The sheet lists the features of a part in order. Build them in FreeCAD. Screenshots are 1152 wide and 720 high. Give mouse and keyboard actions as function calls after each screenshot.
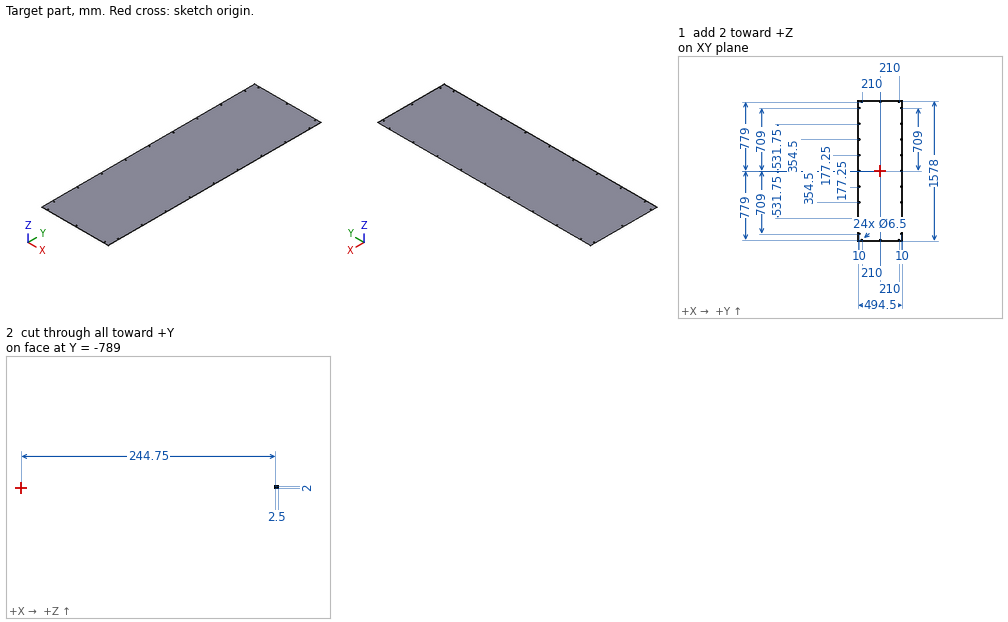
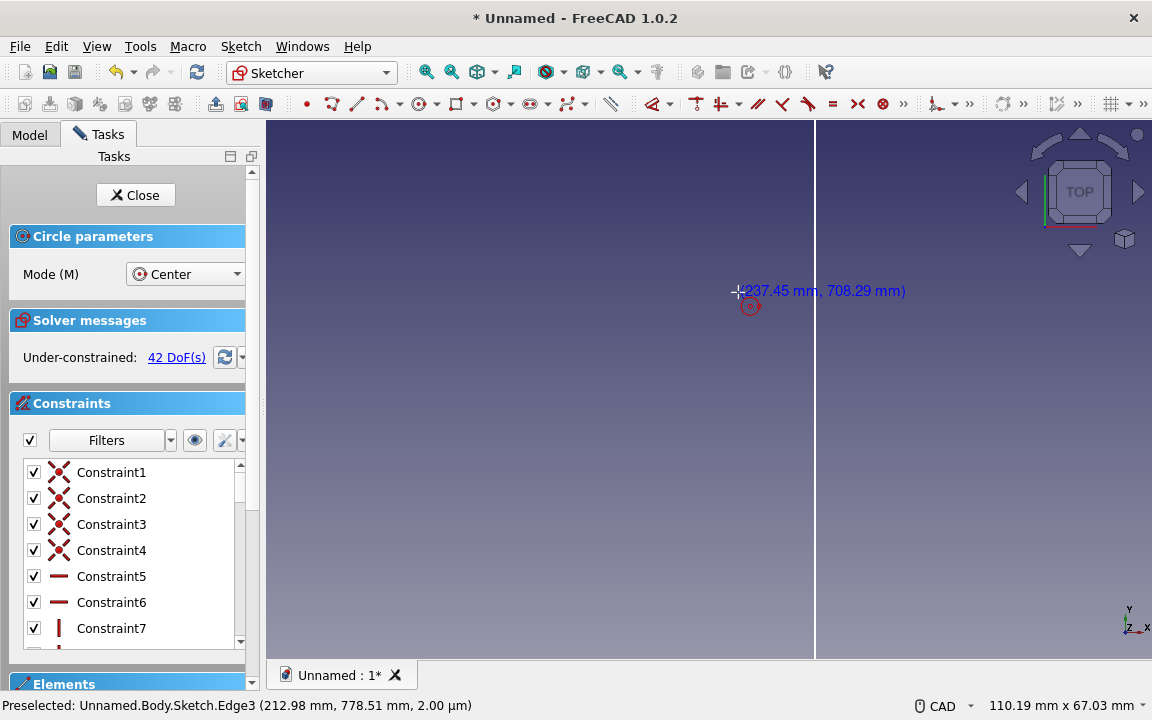
scroll(703, 196, down, 17)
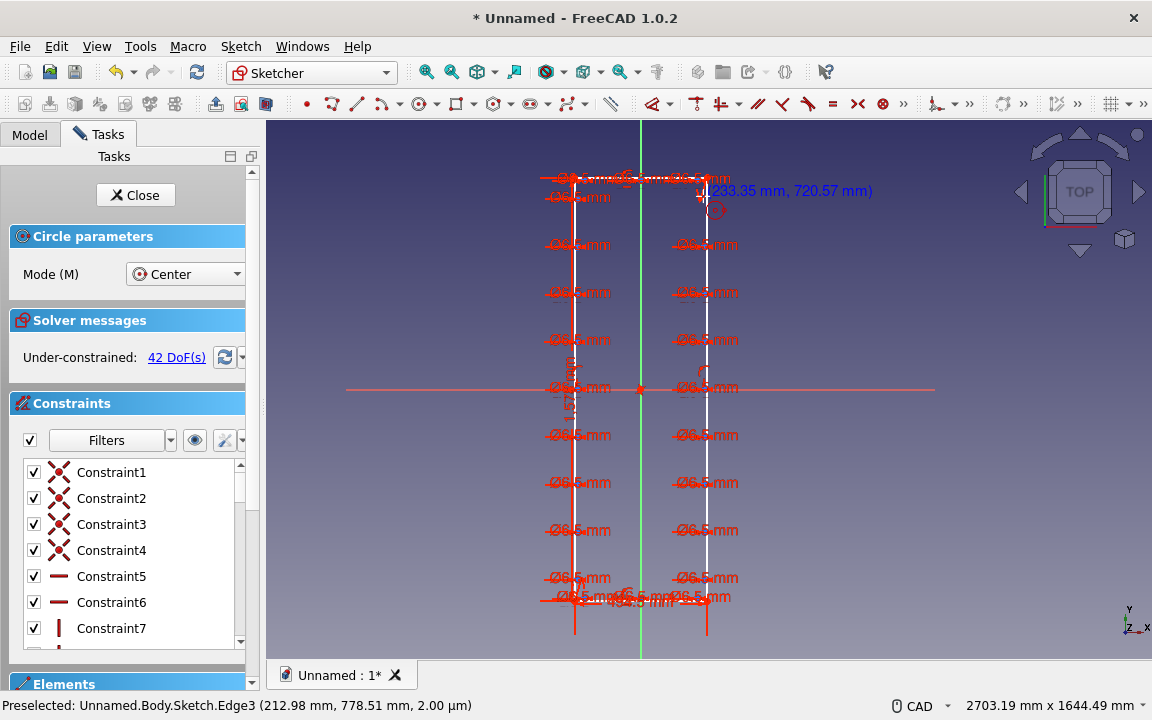
scroll(705, 199, up, 9)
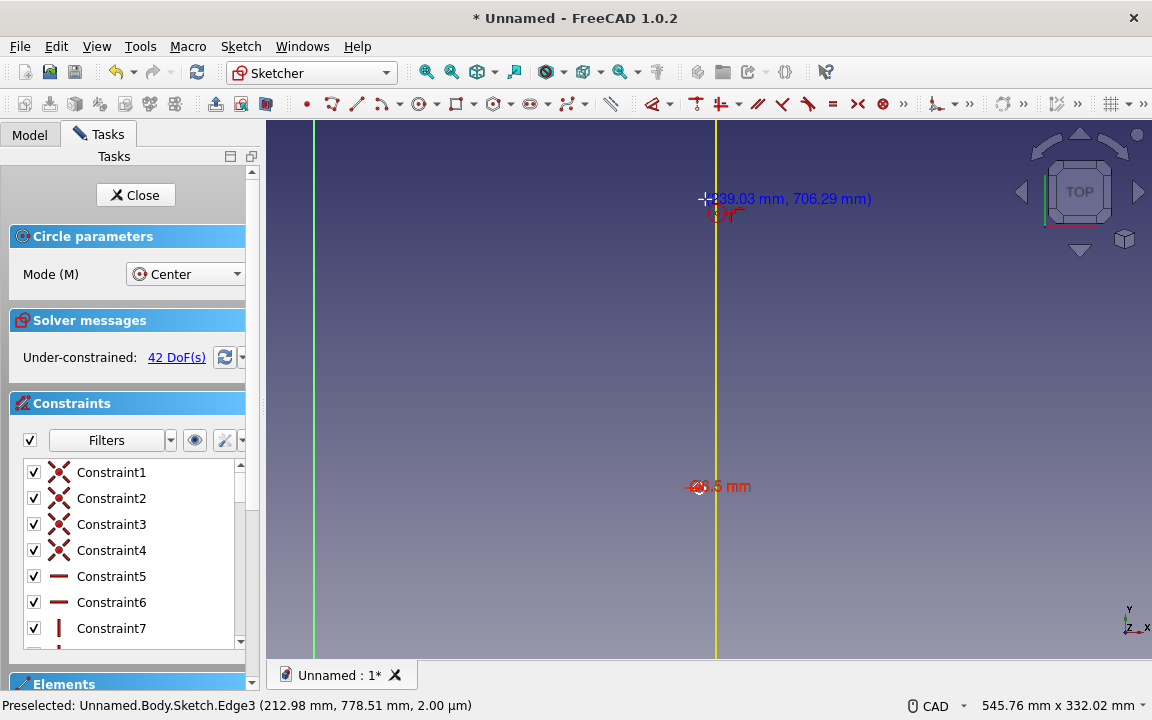
click(700, 200)
move(696, 196)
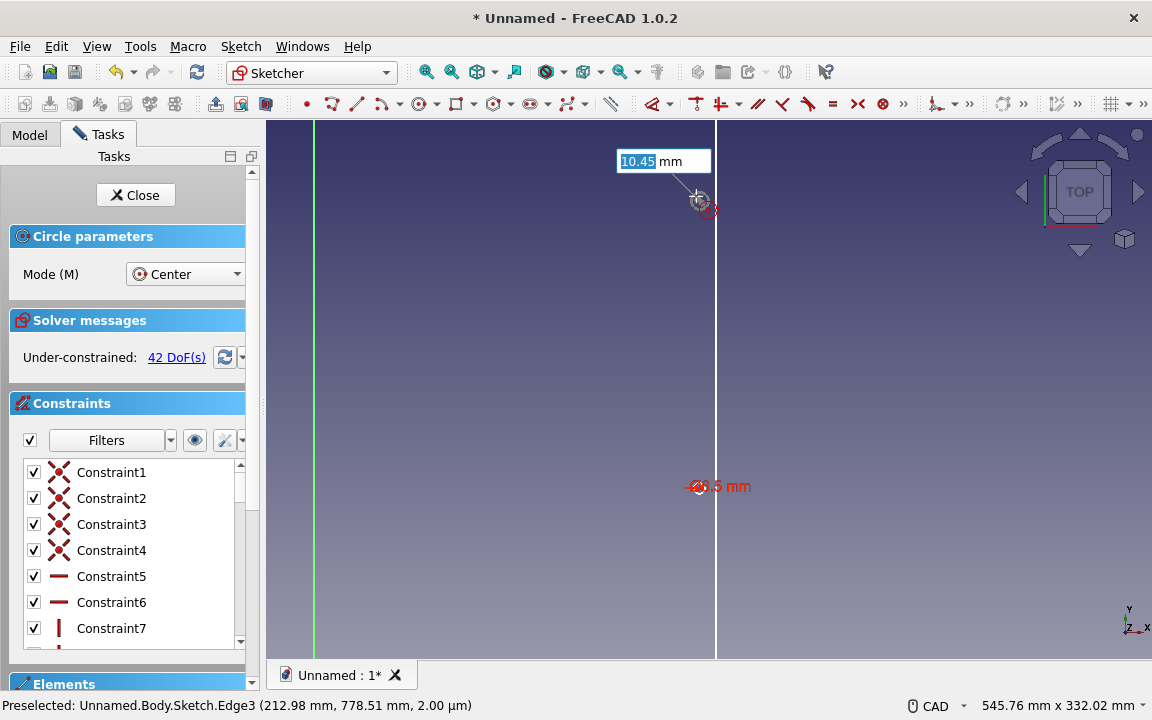
text(6.5)
key(Return)
key(Escape)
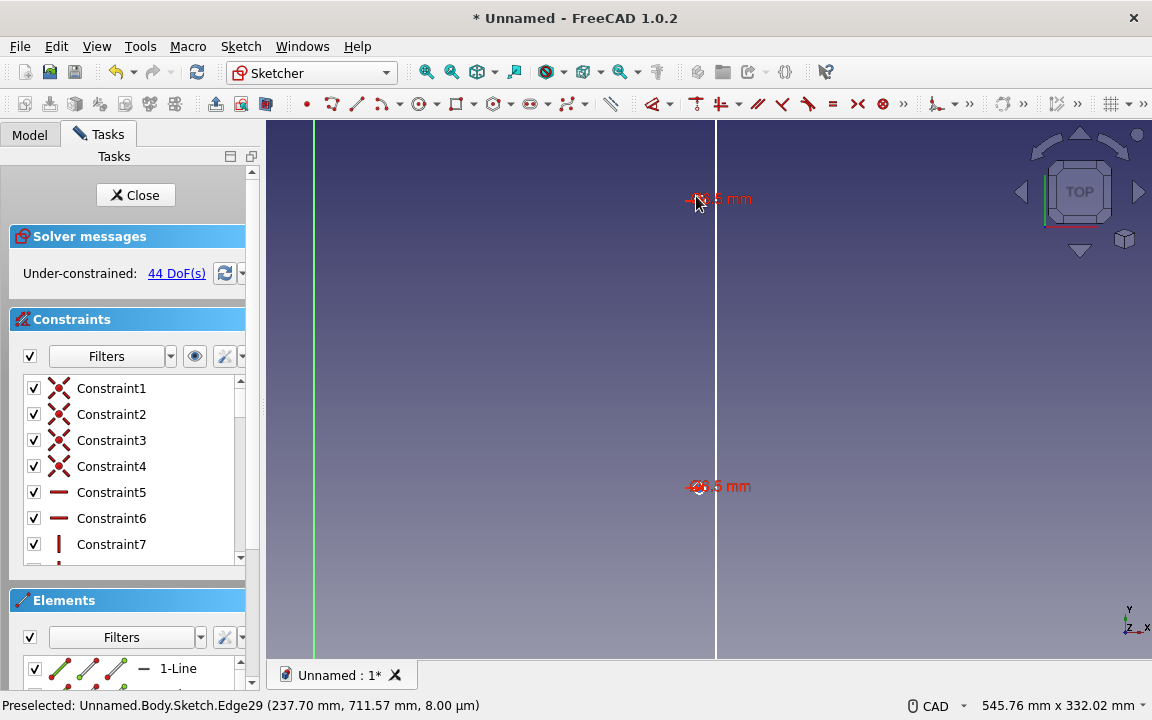
scroll(692, 239, down, 10)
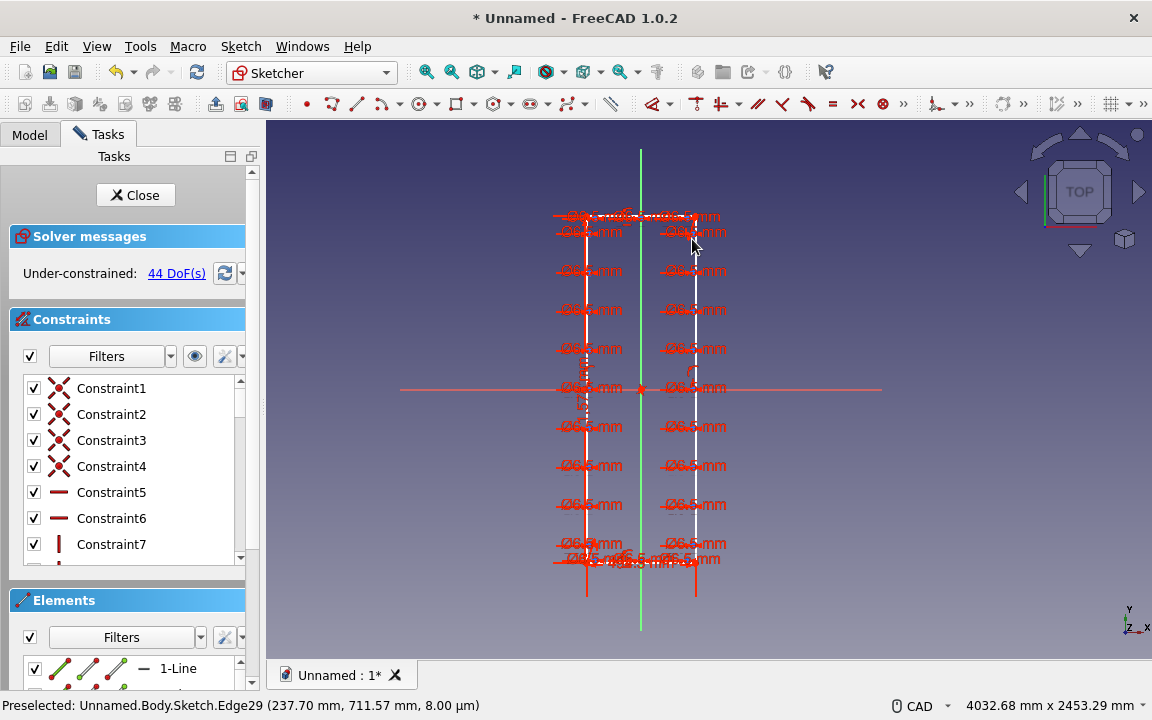
click(589, 546)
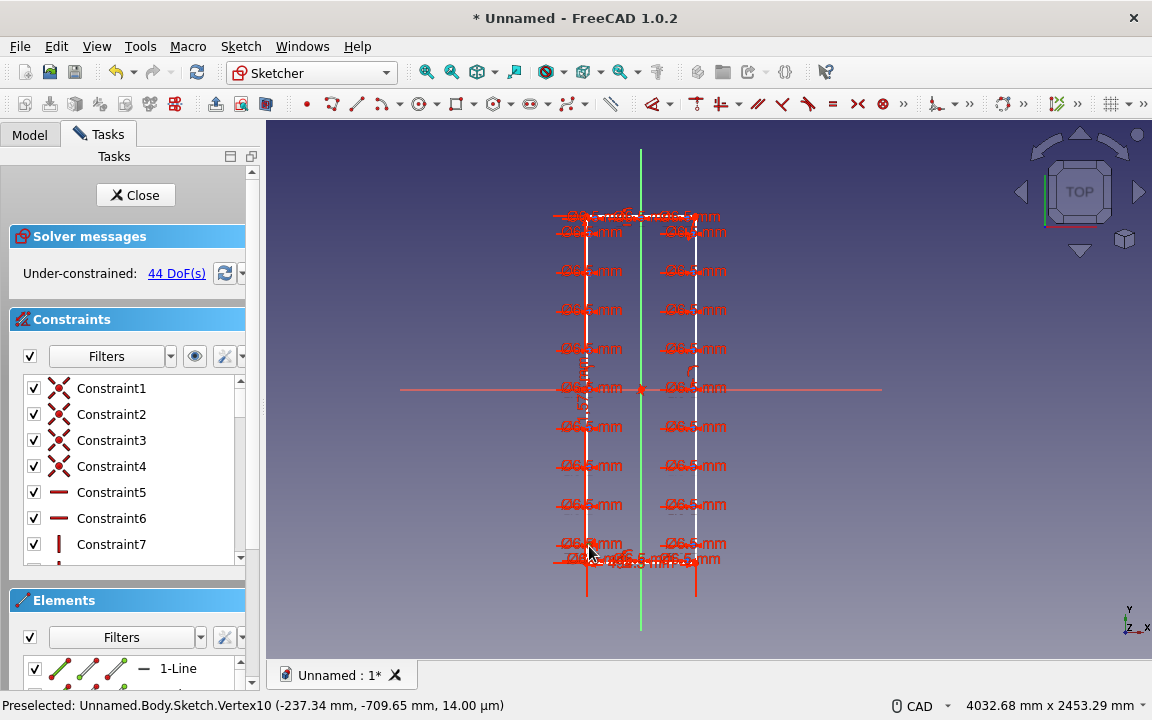
click(589, 507)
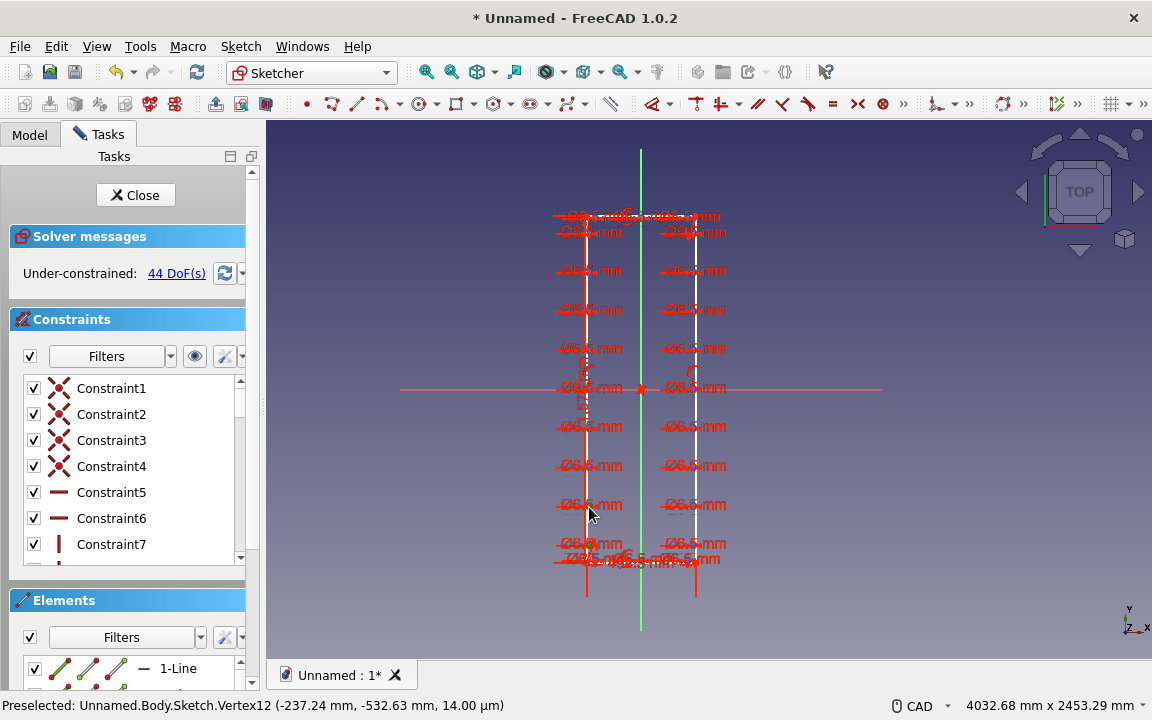
key(v)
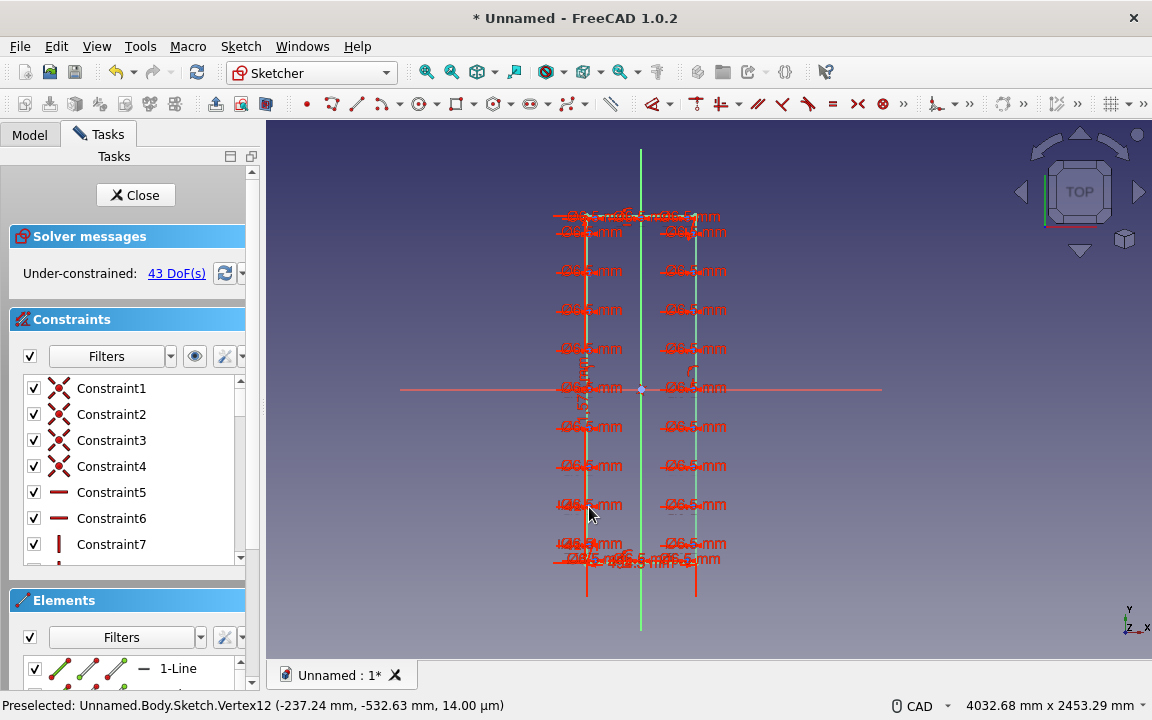
click(589, 507)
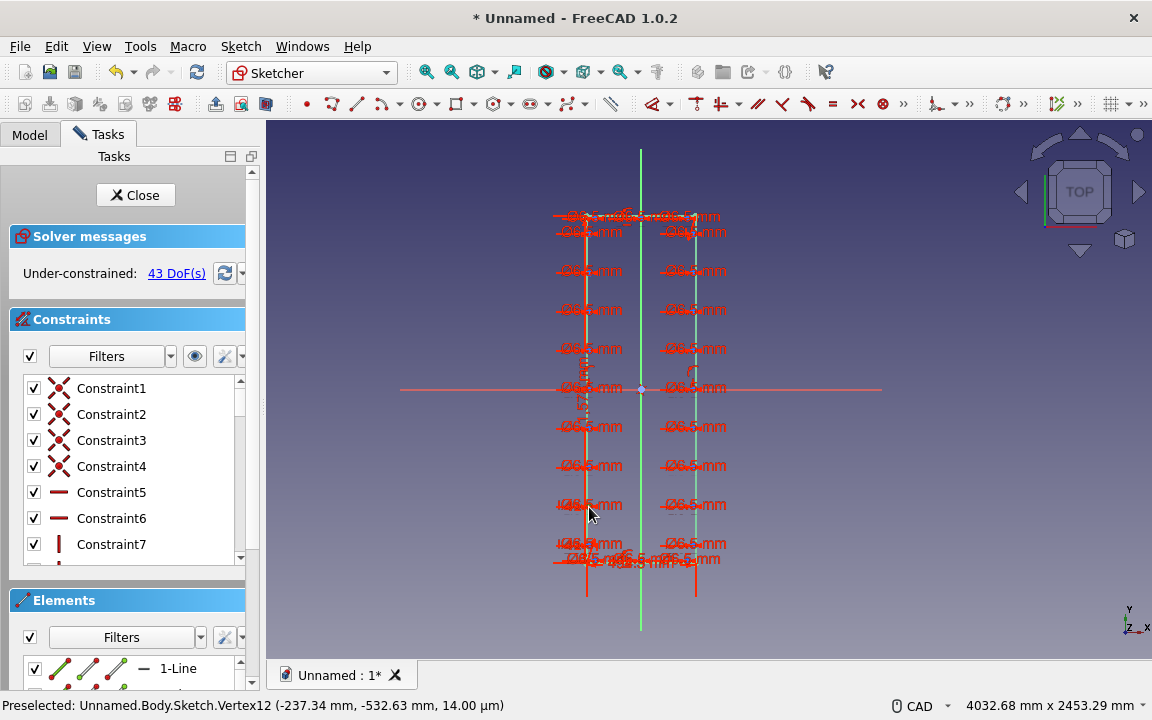
click(589, 468)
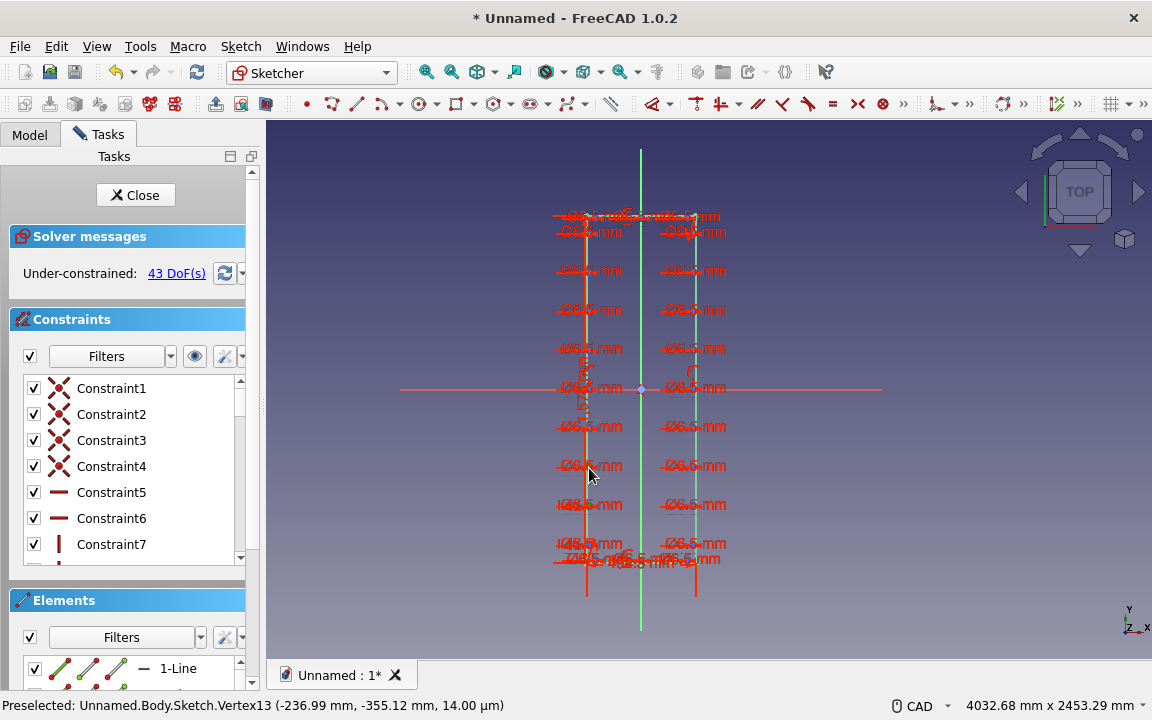
click(738, 104)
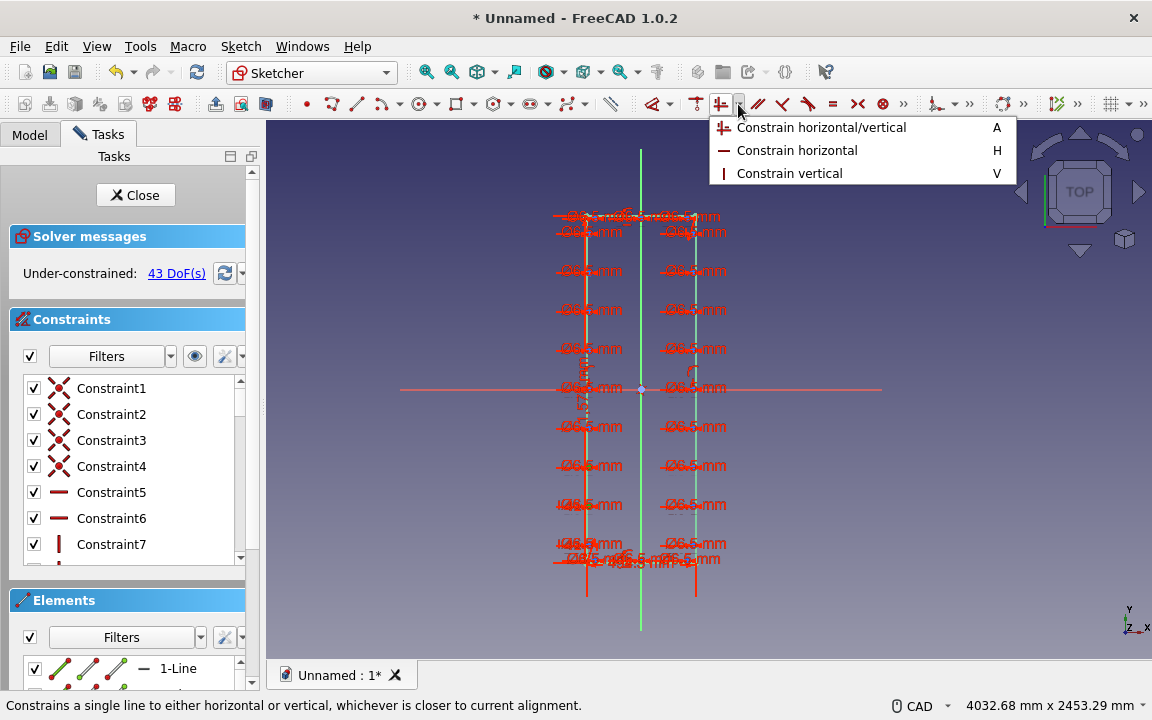
click(863, 174)